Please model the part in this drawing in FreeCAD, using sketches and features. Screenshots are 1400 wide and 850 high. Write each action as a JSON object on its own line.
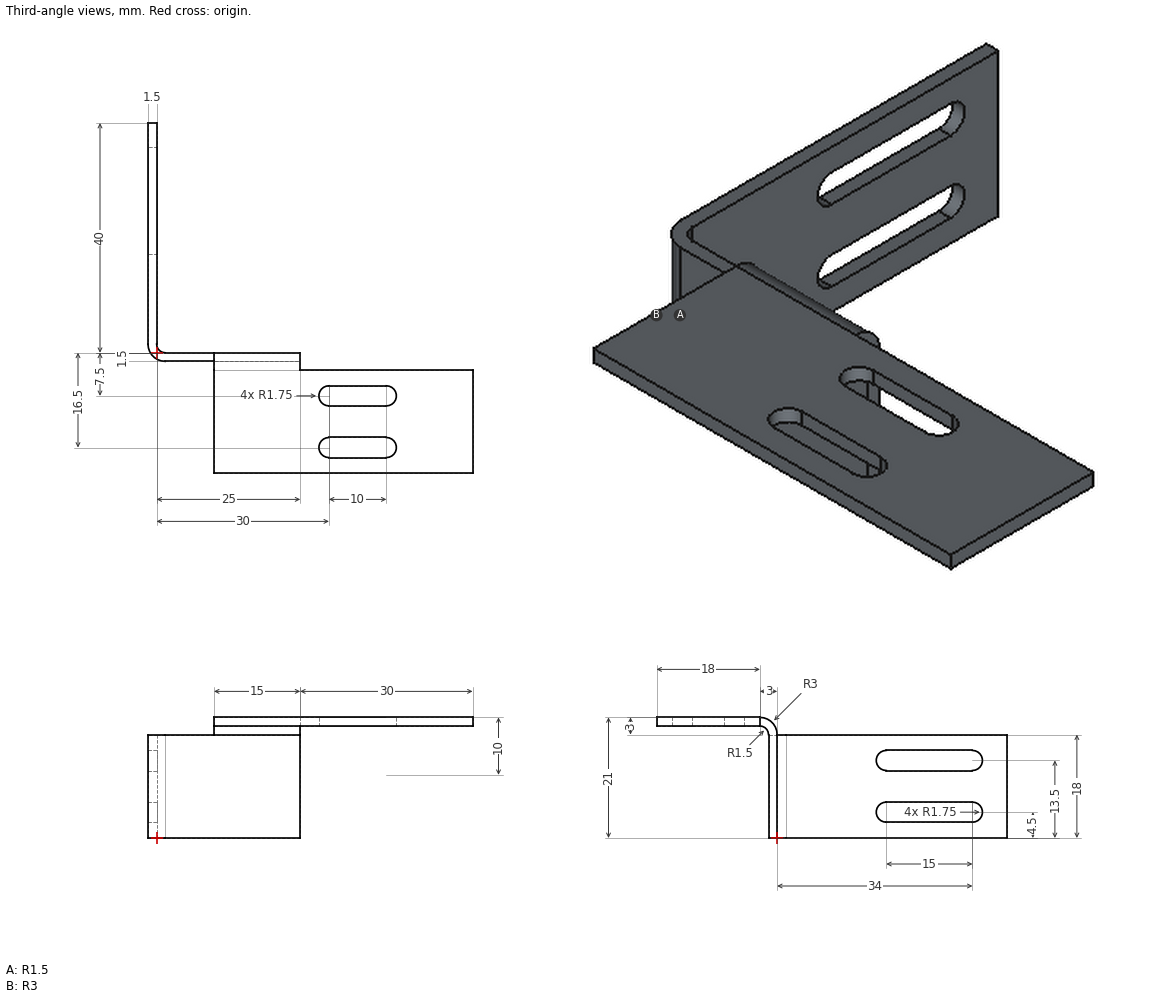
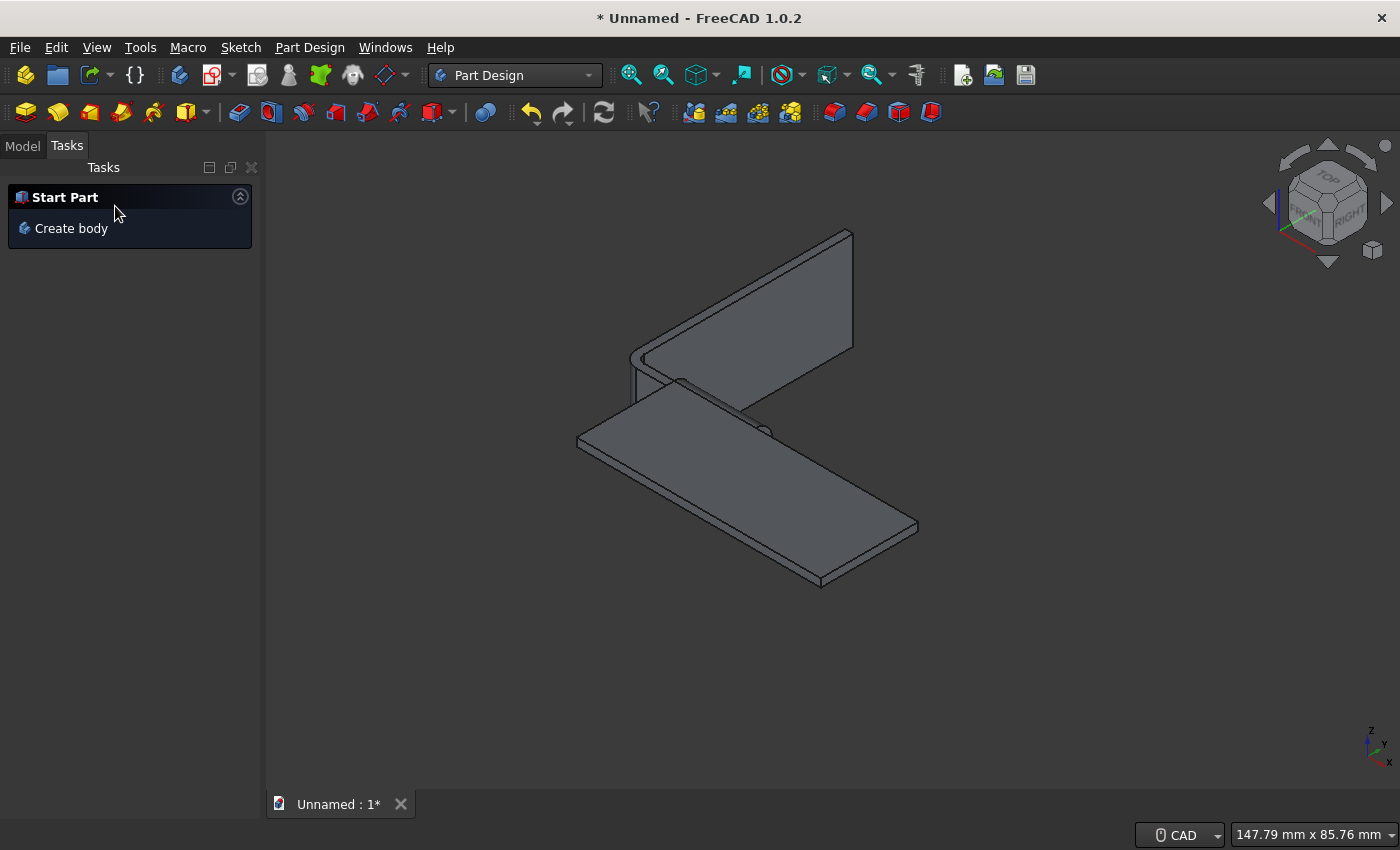
{"action": "key", "text": "6"}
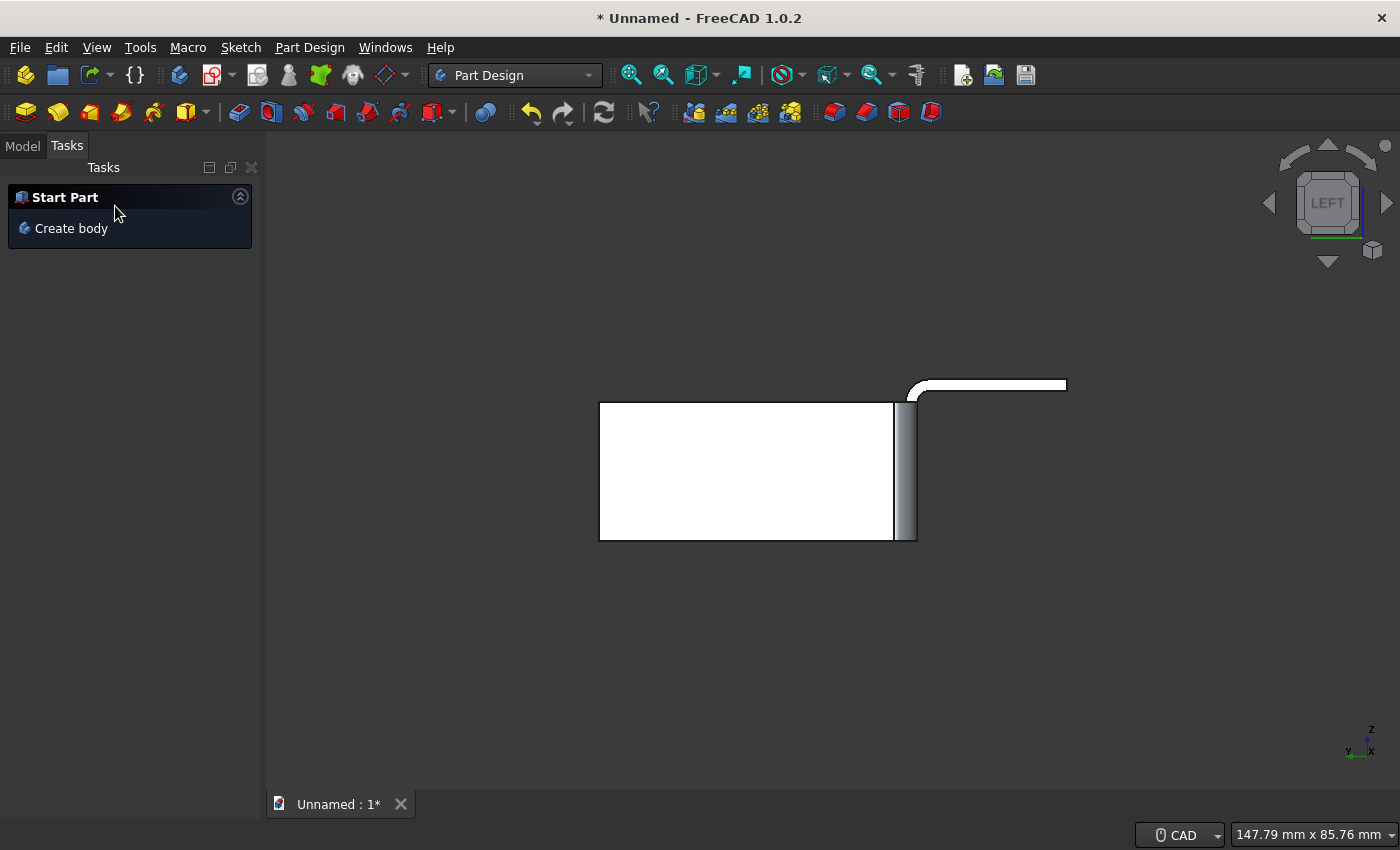
{"action": "key", "text": "v f"}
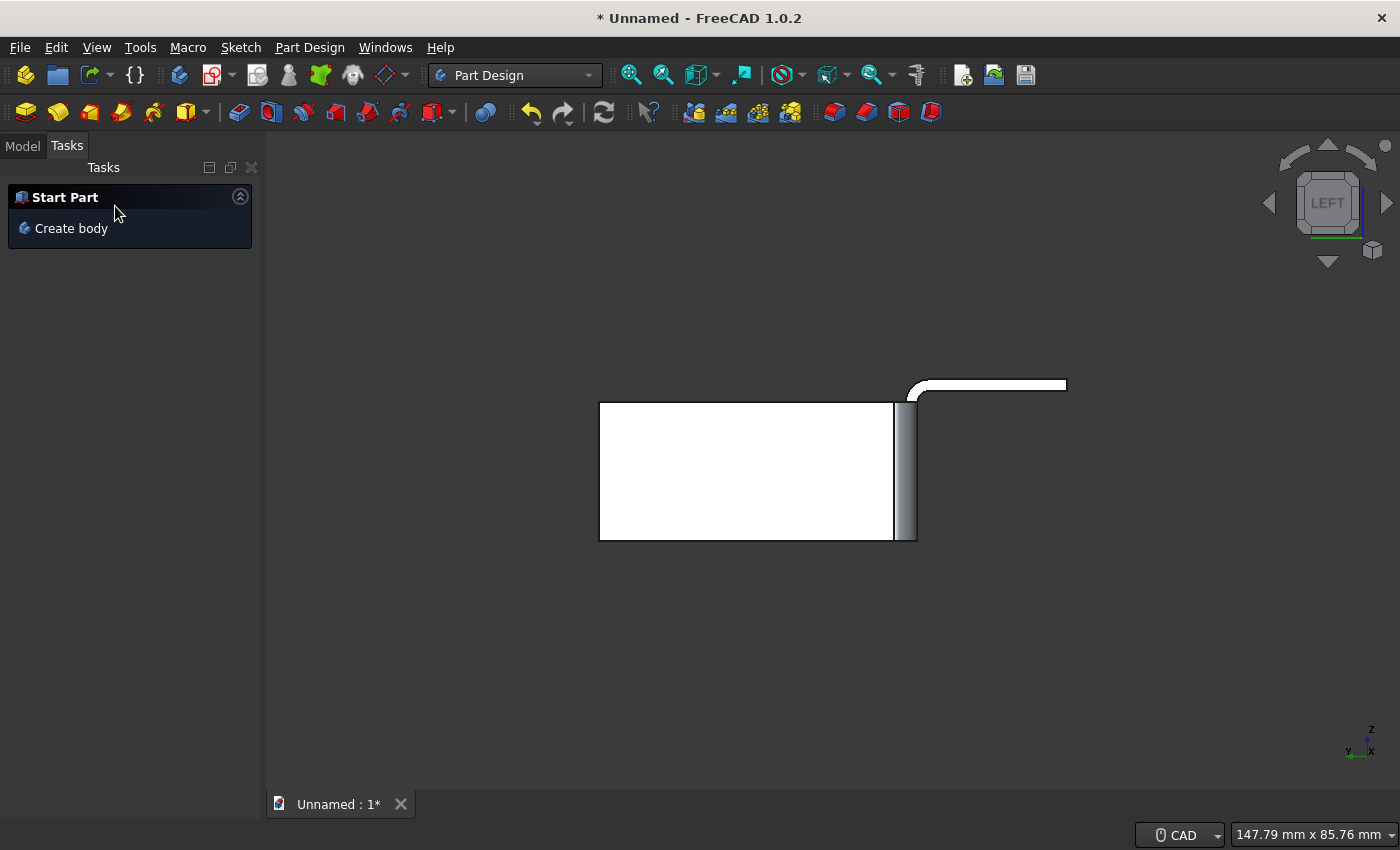
{"action": "left_click", "coordinate": [704, 471]}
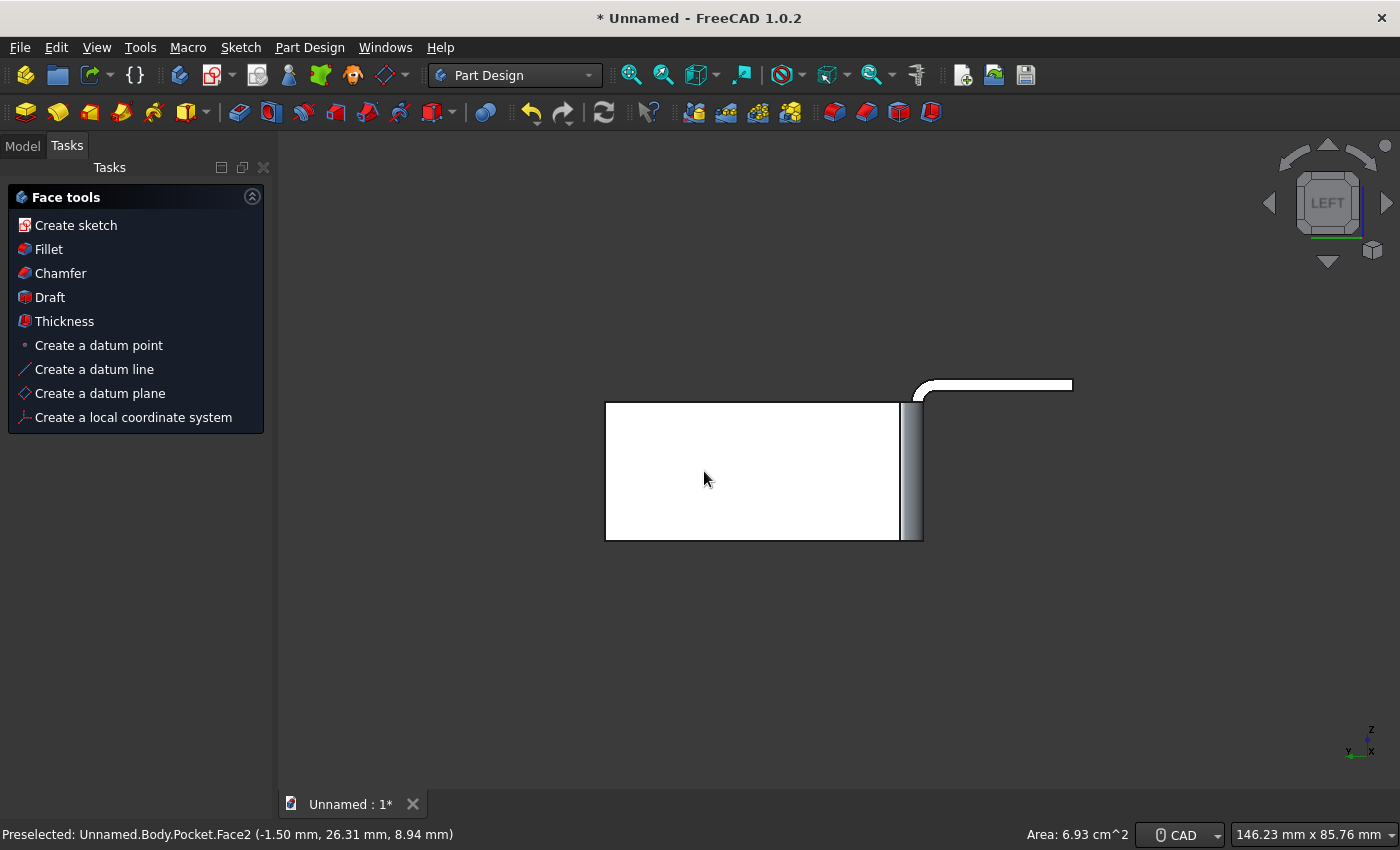
{"action": "left_click", "coordinate": [212, 76]}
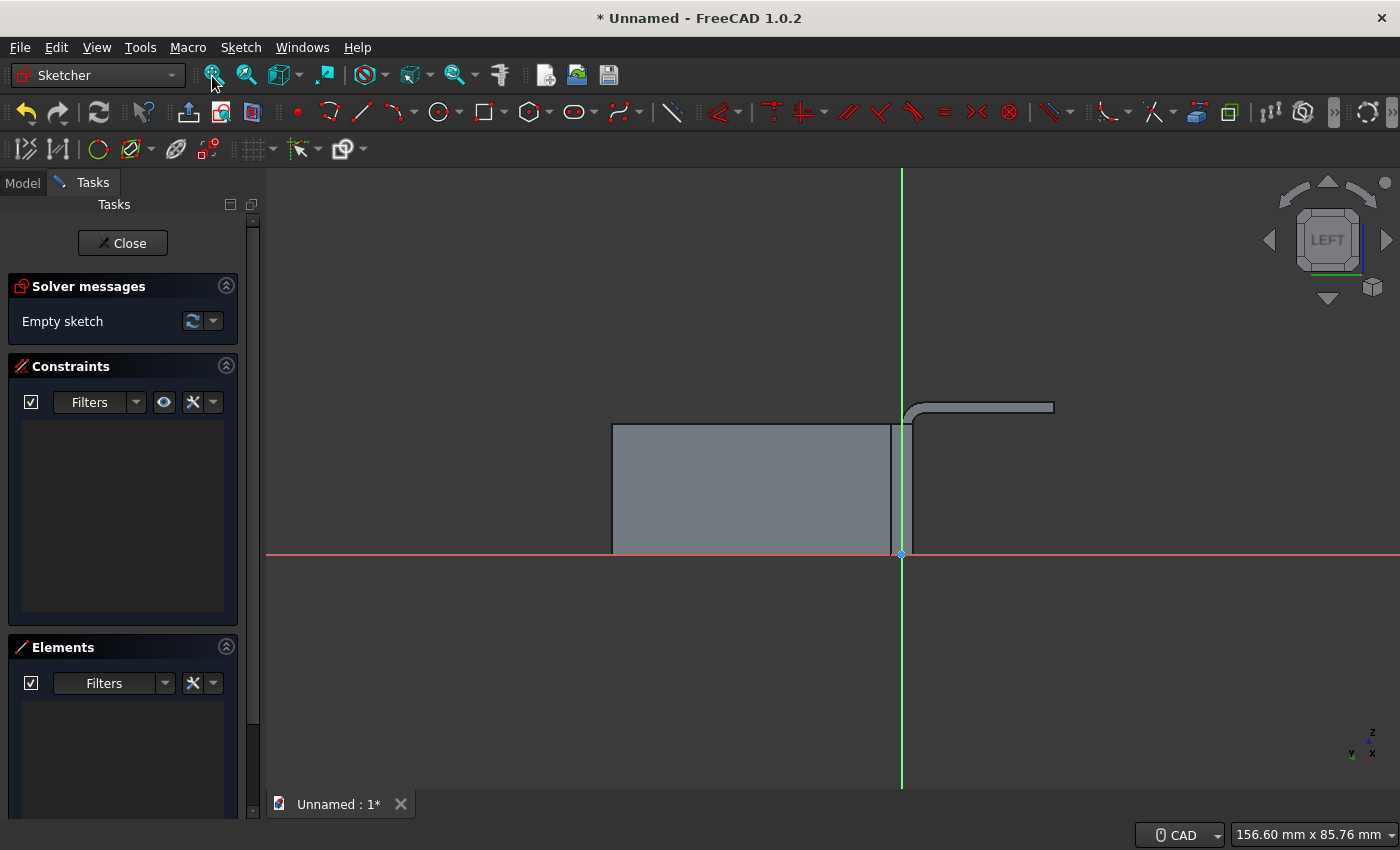
{"action": "scroll", "coordinate": [777, 511], "scroll_direction": "up", "scroll_amount": 5}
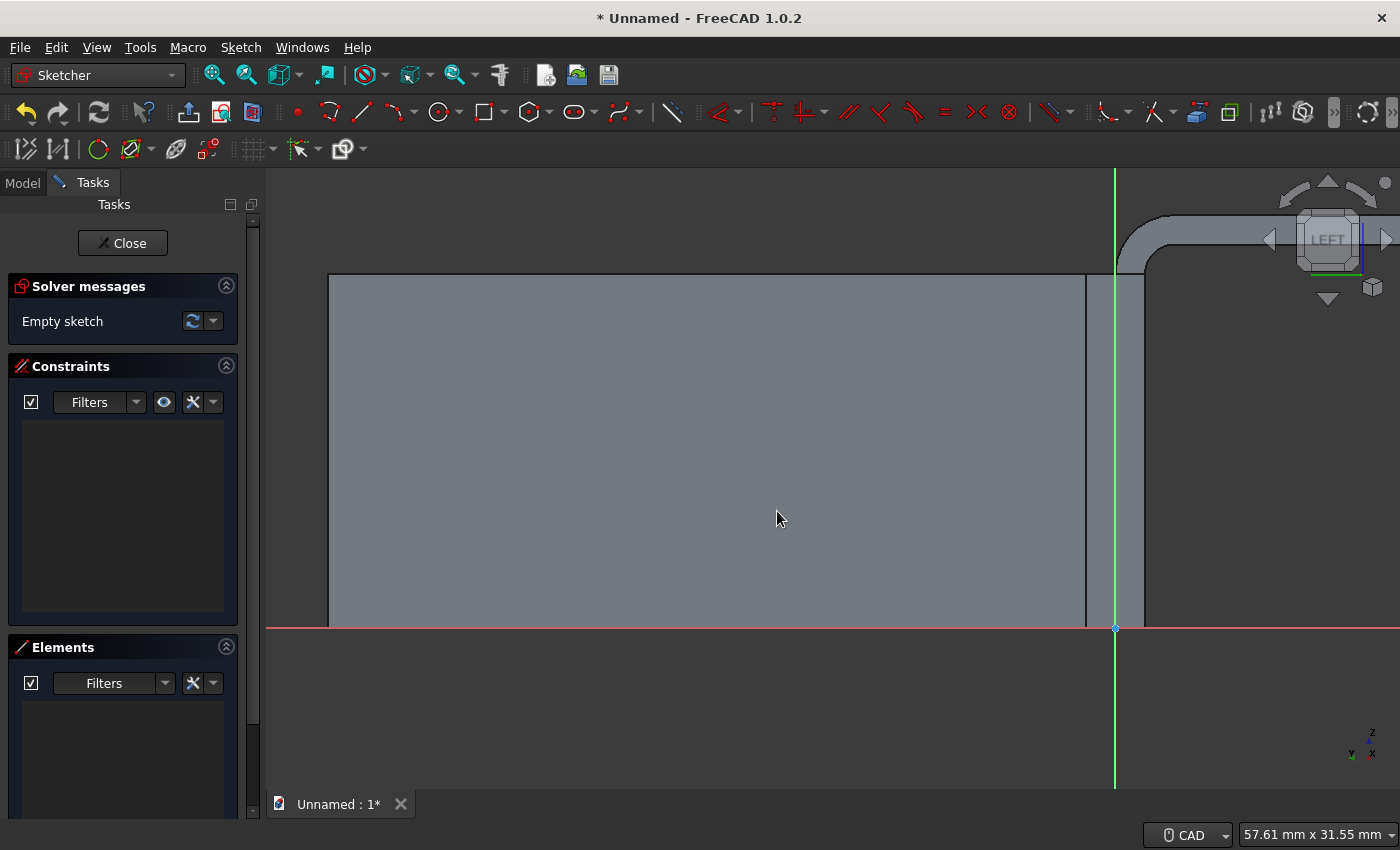
{"action": "key", "text": "g s"}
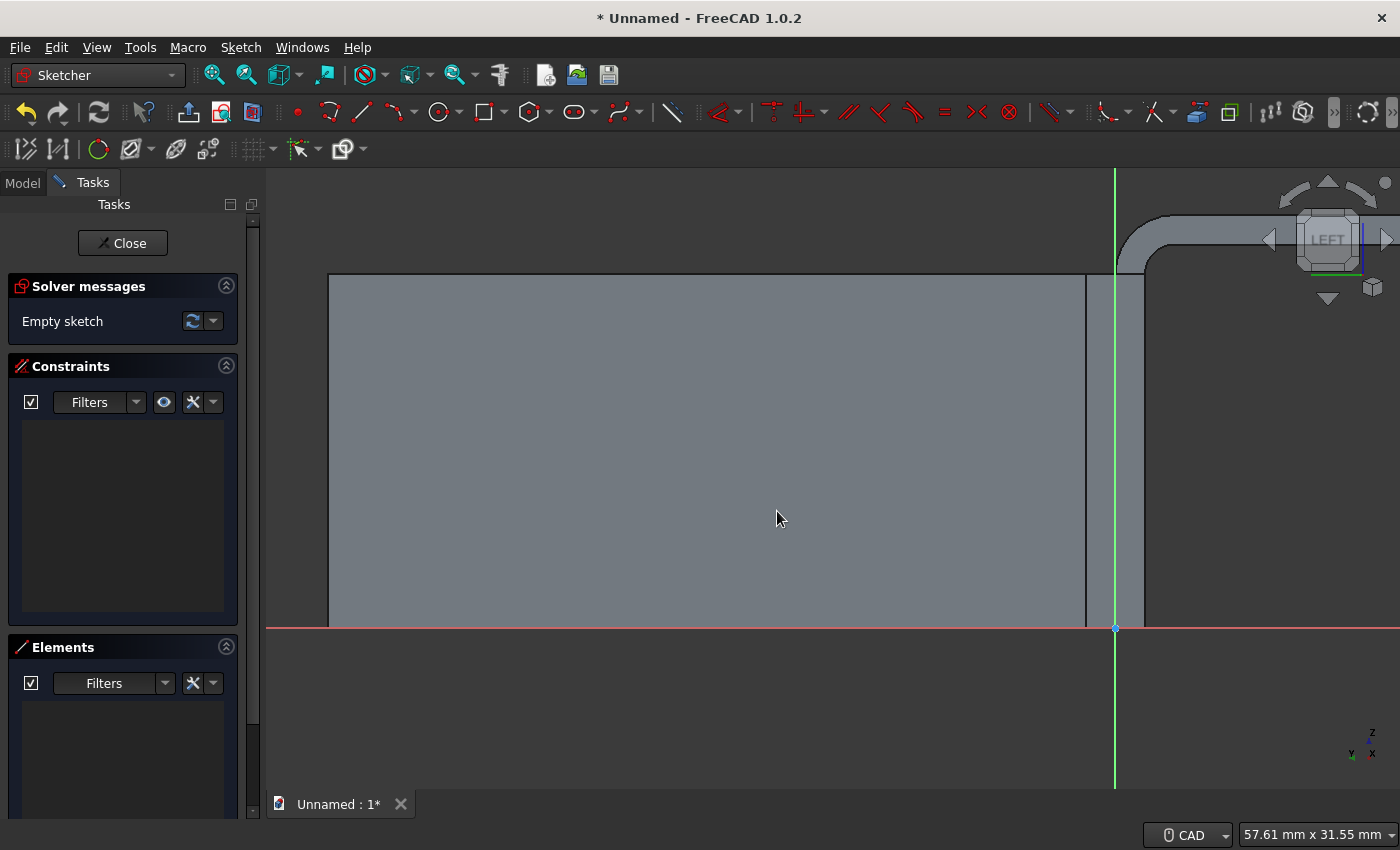
{"action": "left_click", "coordinate": [446, 540]}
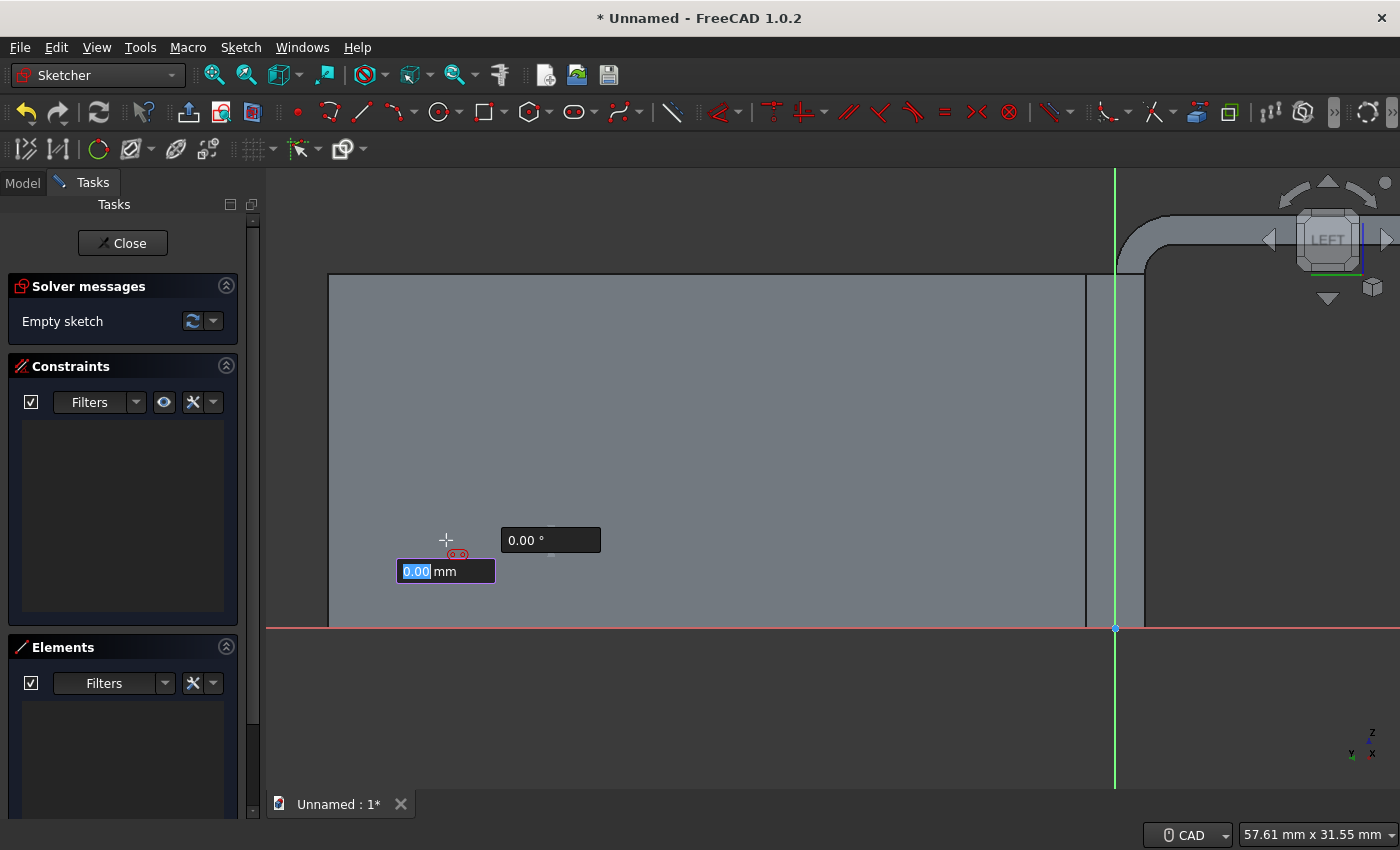
{"action": "left_click", "coordinate": [741, 540]}